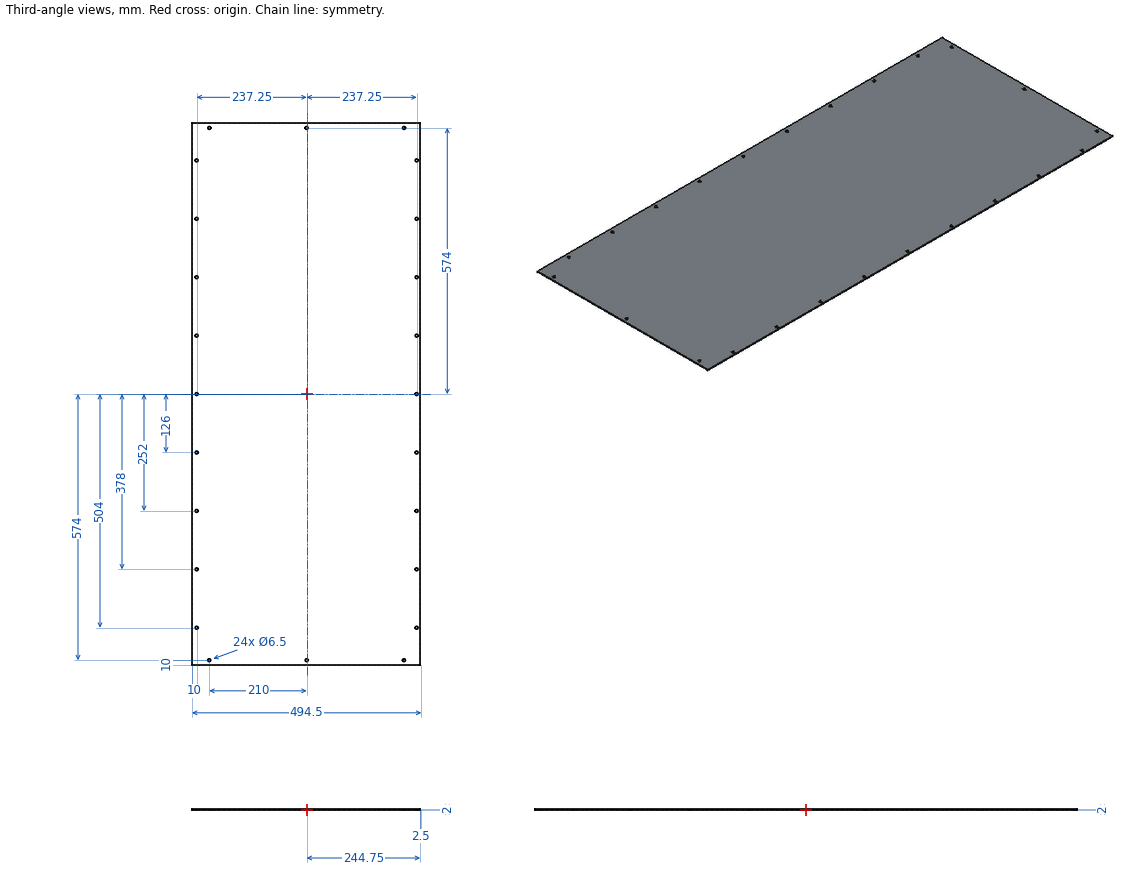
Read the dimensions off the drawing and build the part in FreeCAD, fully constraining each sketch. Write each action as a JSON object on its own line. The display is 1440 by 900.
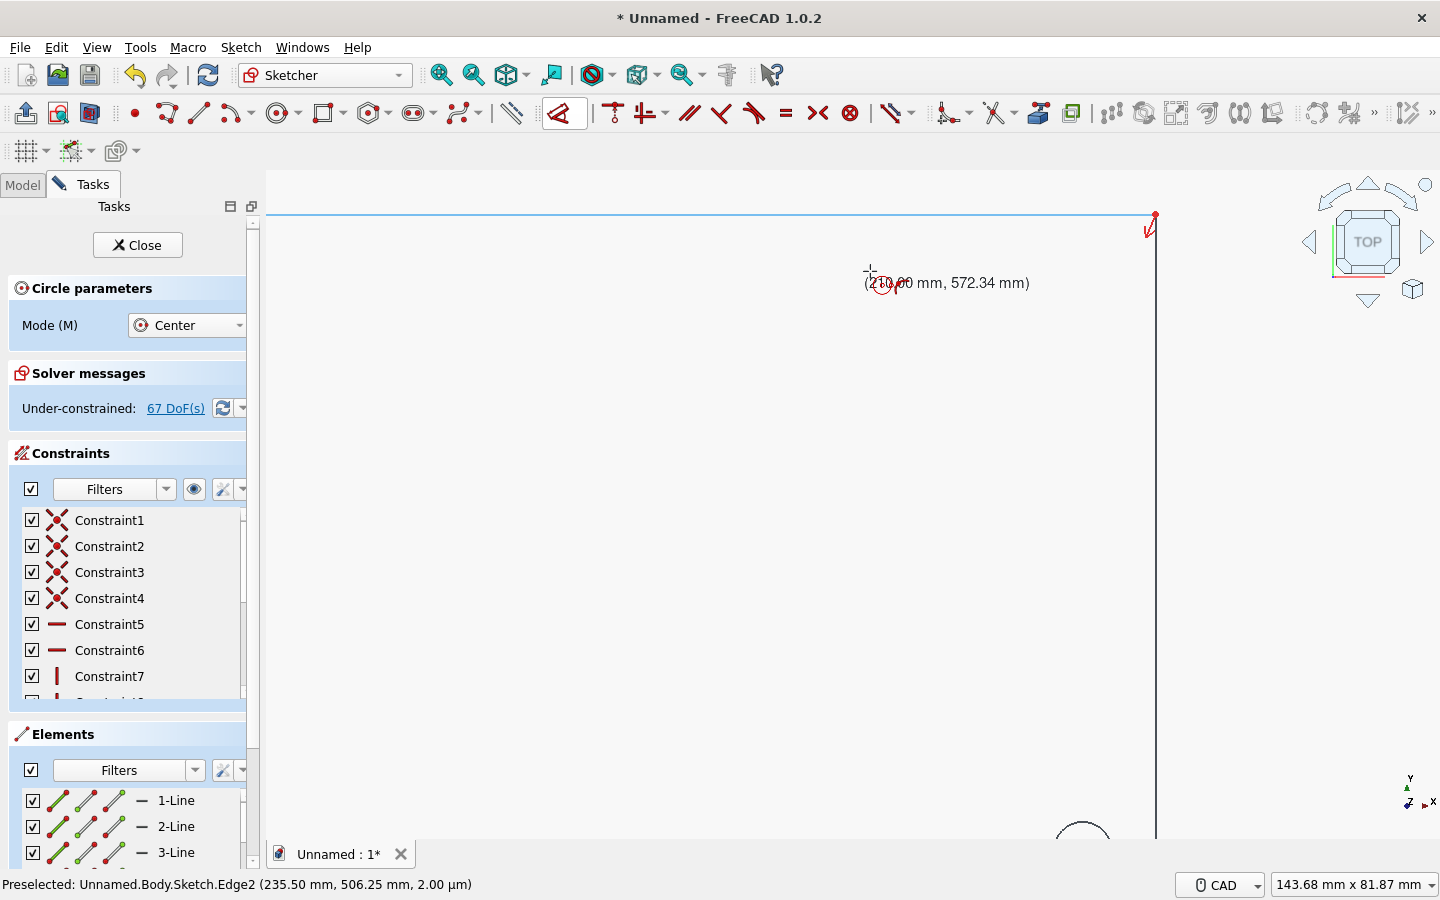
{"action": "scroll", "coordinate": [870, 271], "scroll_direction": "down", "scroll_amount": 15}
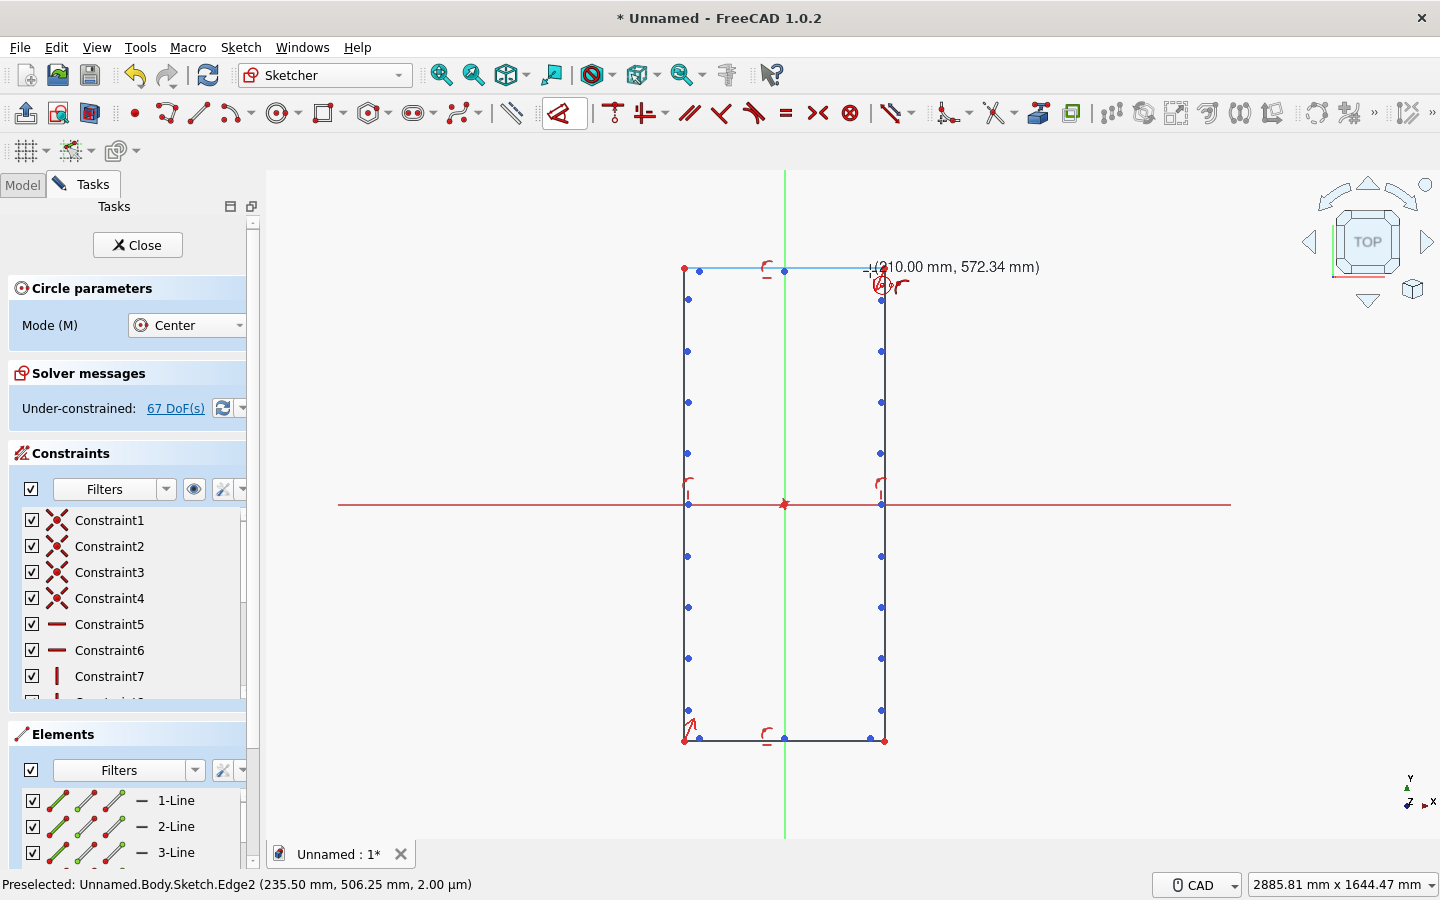
{"action": "scroll", "coordinate": [870, 271], "scroll_direction": "up", "scroll_amount": 7}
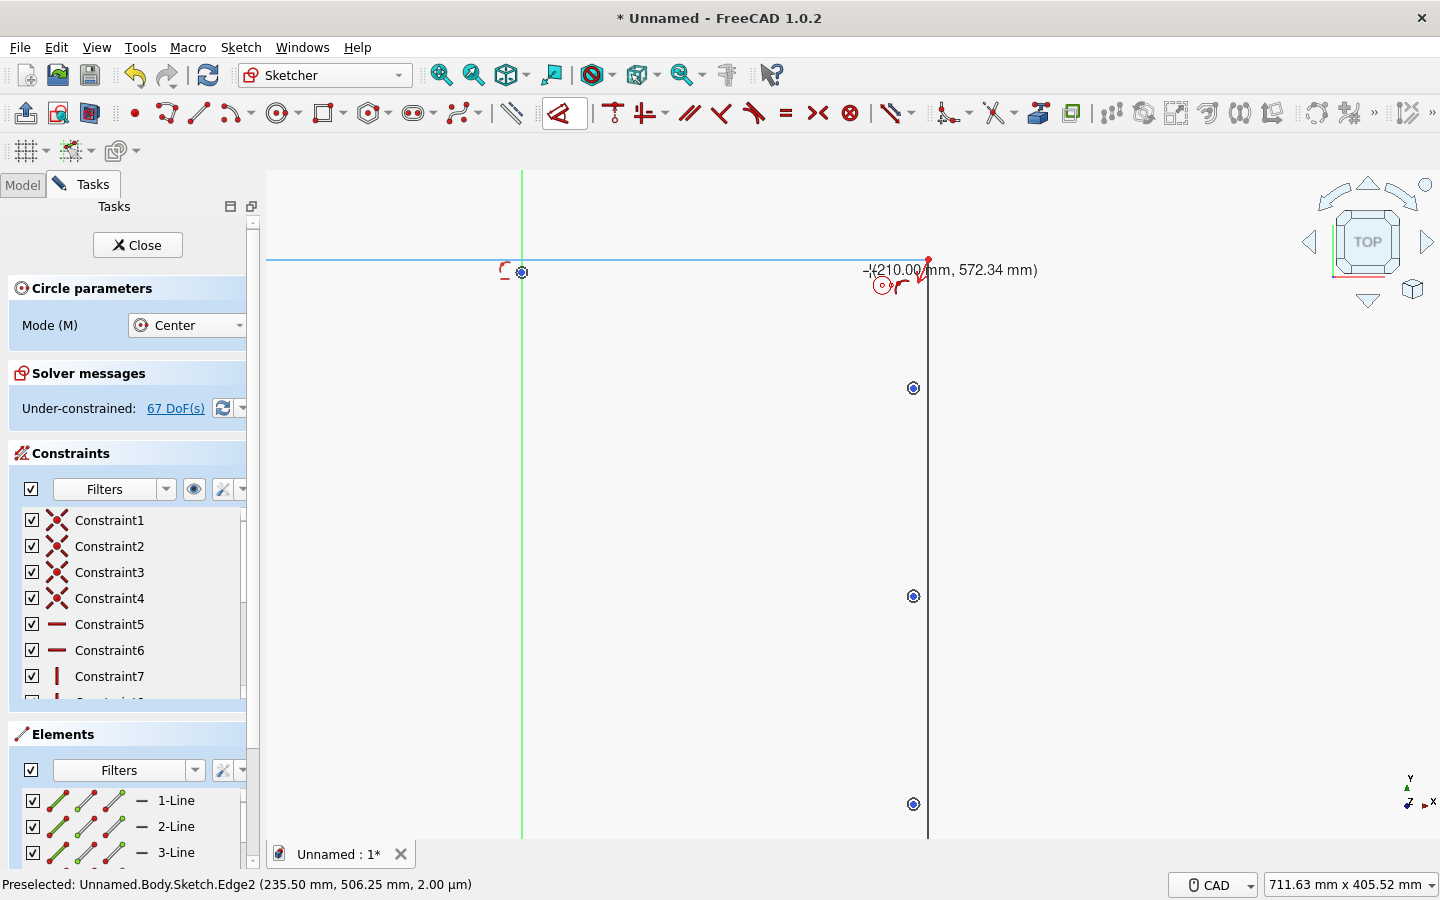
{"action": "left_click", "coordinate": [868, 272]}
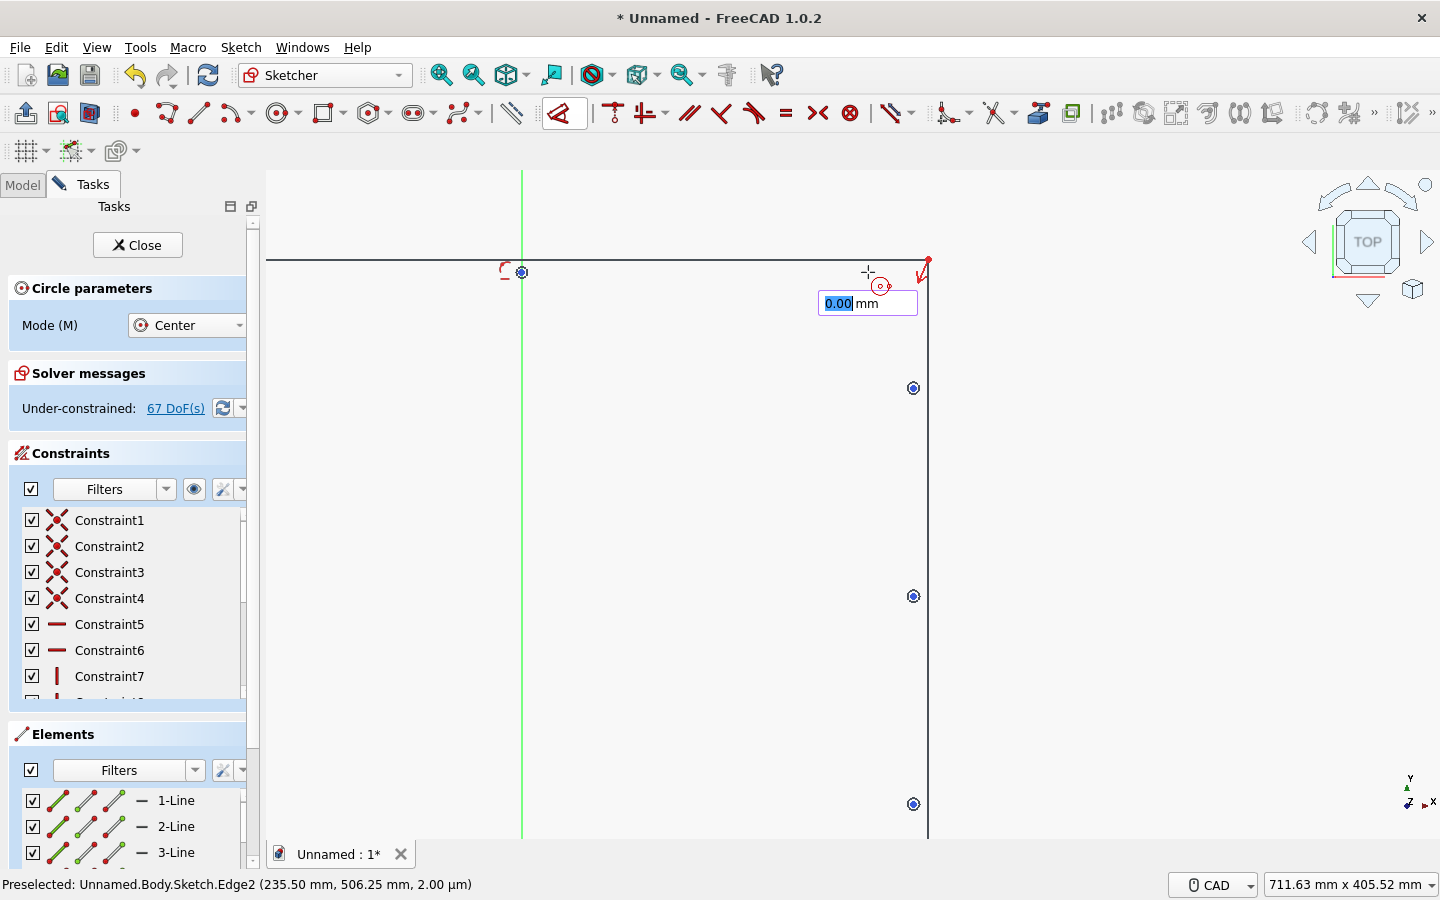
{"action": "scroll", "coordinate": [872, 276], "scroll_direction": "up", "scroll_amount": 6}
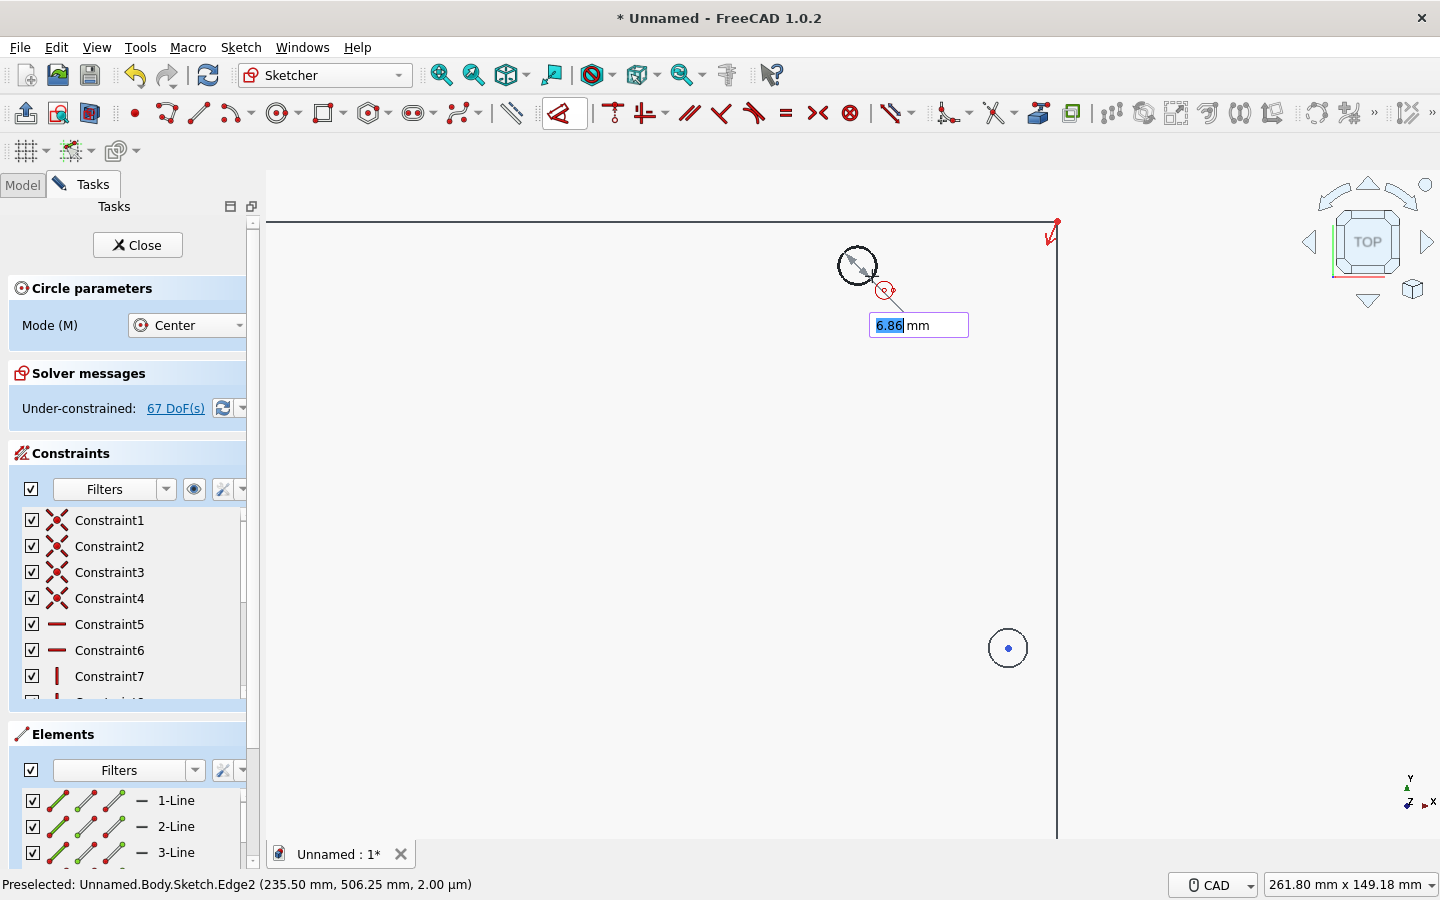
{"action": "left_click", "coordinate": [872, 274]}
{"action": "key", "text": "Escape"}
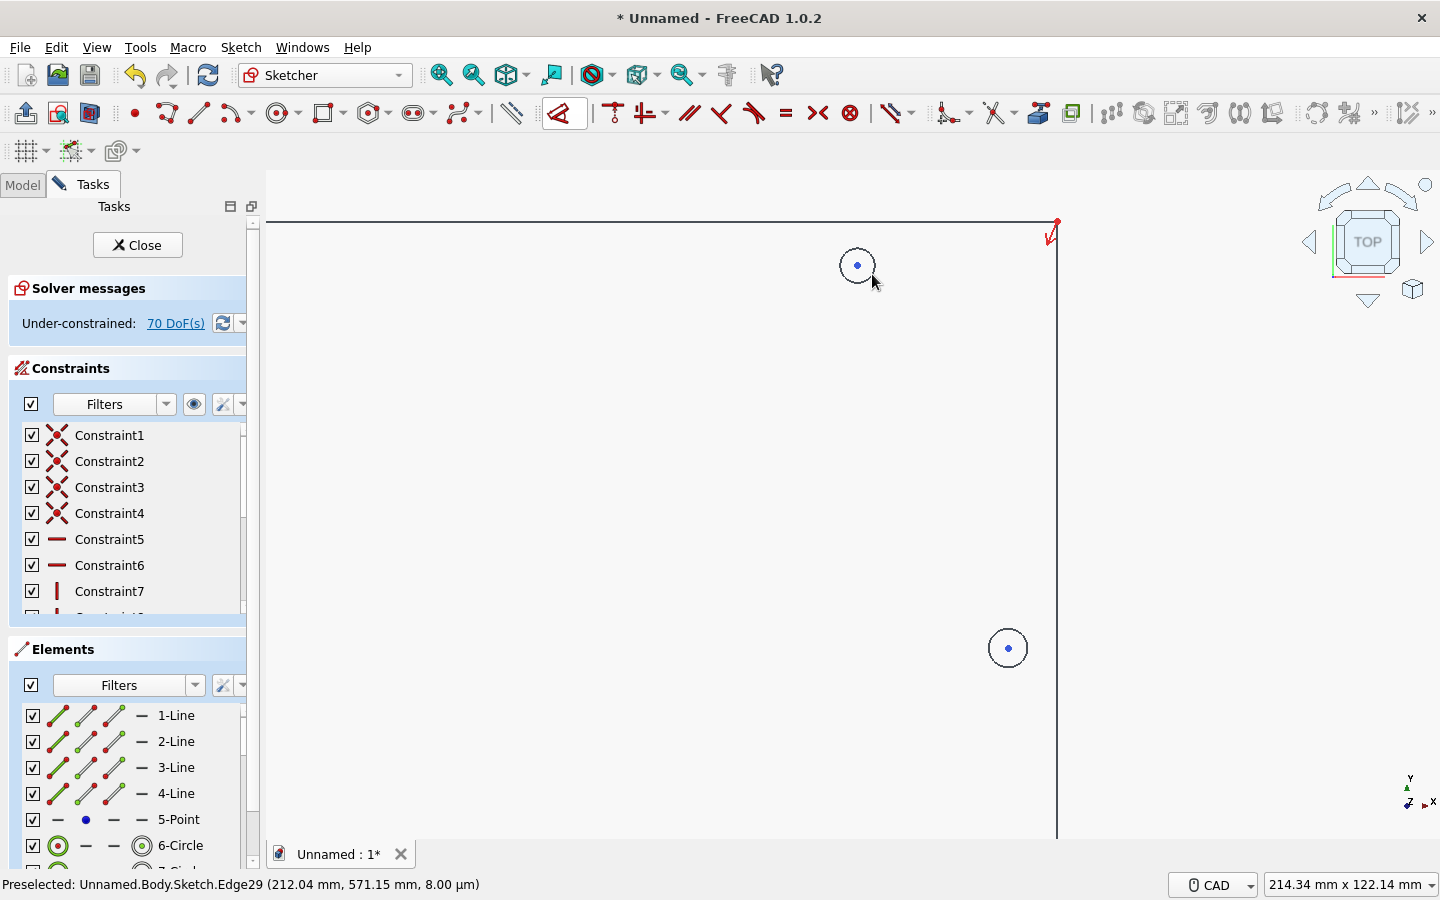
{"action": "scroll", "coordinate": [871, 272], "scroll_direction": "down", "scroll_amount": 13}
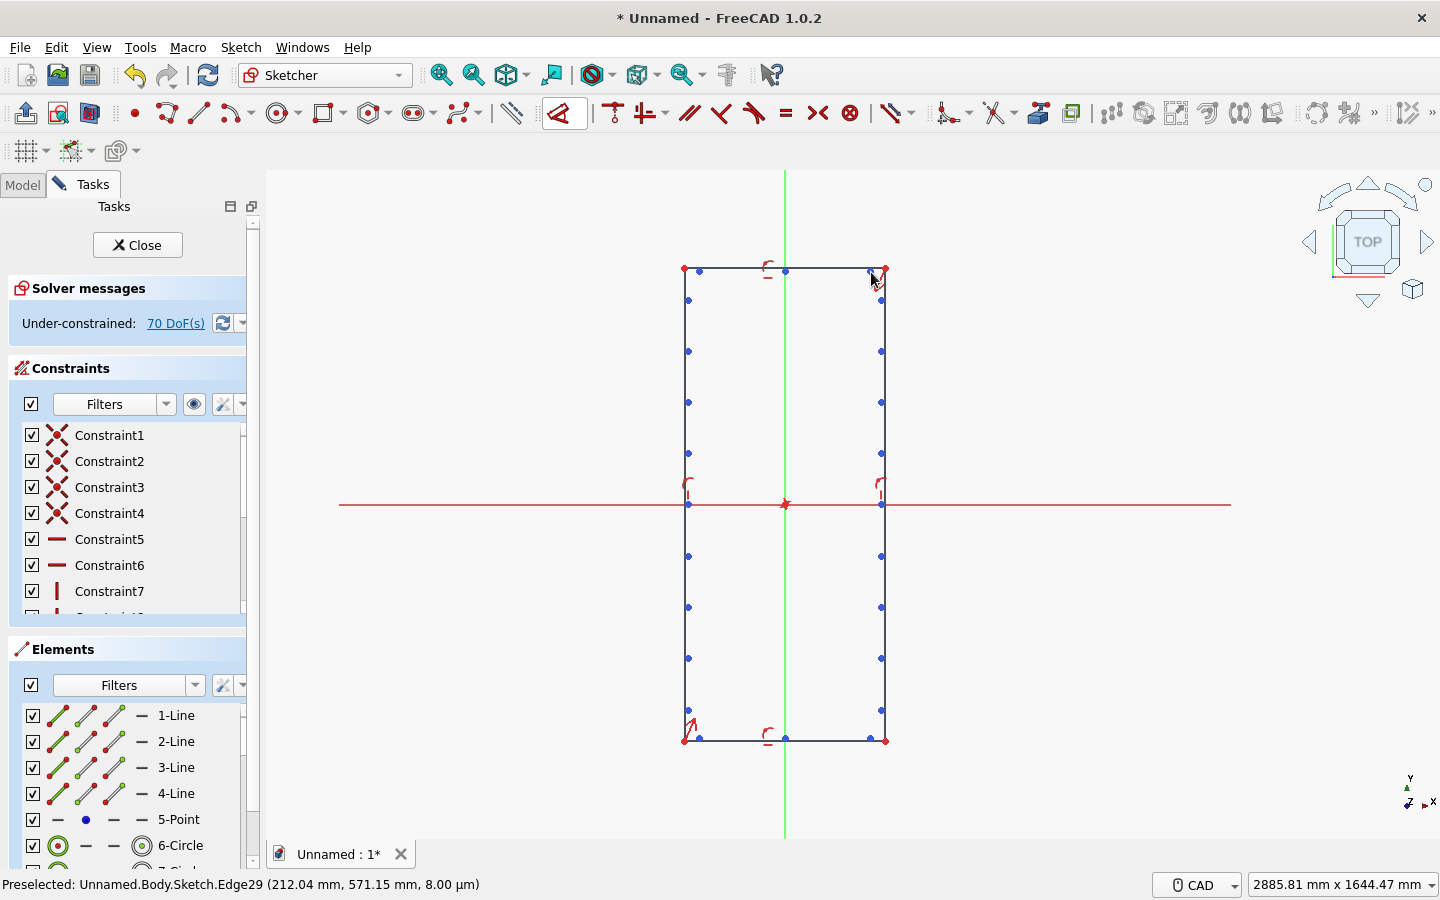
{"action": "scroll", "coordinate": [701, 738], "scroll_direction": "up", "scroll_amount": 12}